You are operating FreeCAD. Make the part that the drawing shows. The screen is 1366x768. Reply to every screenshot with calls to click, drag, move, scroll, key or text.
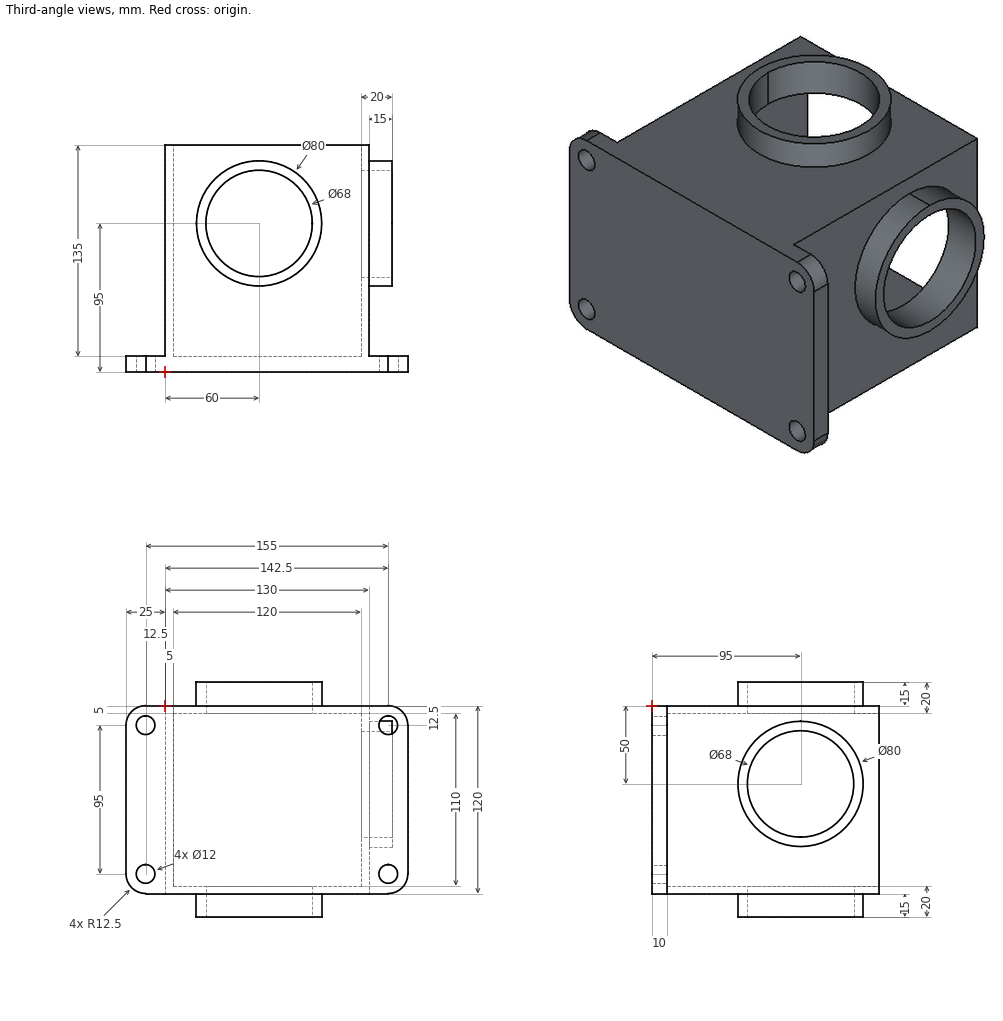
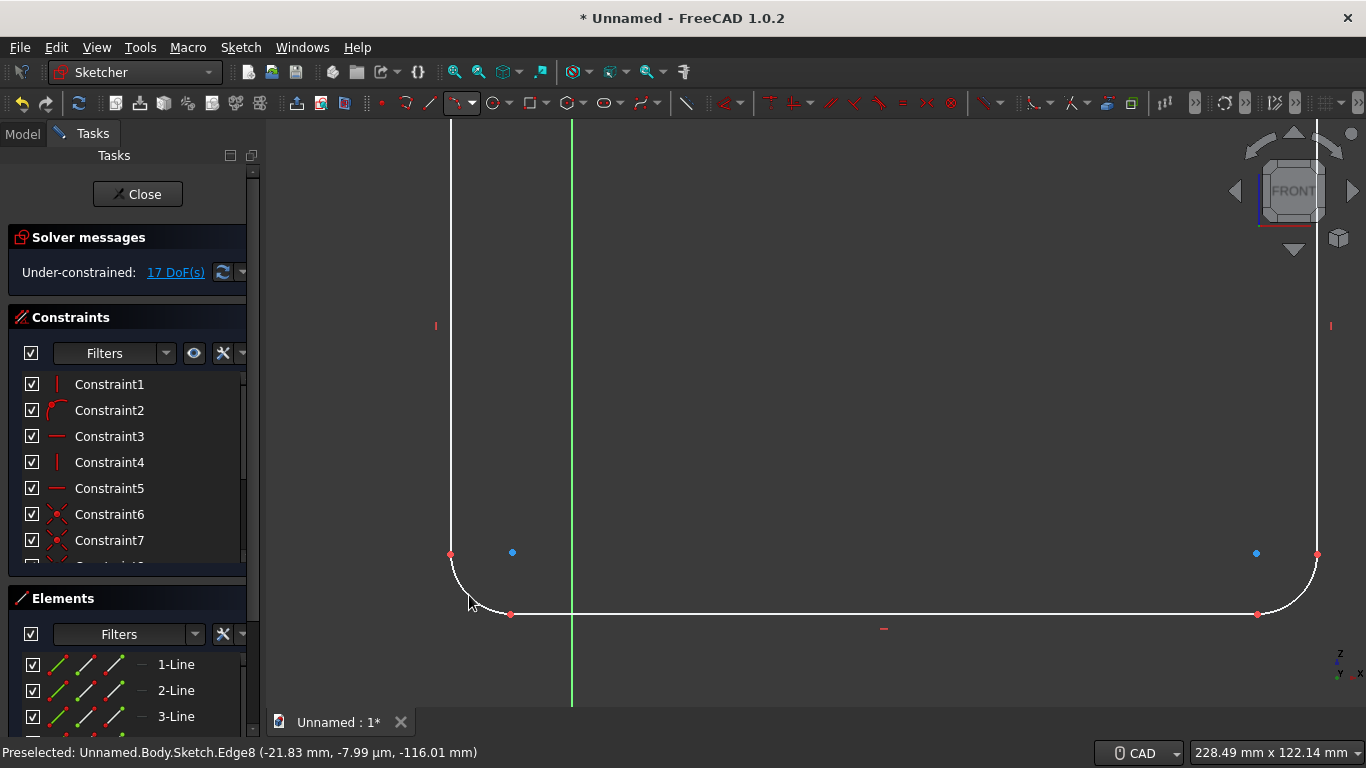
click(451, 417)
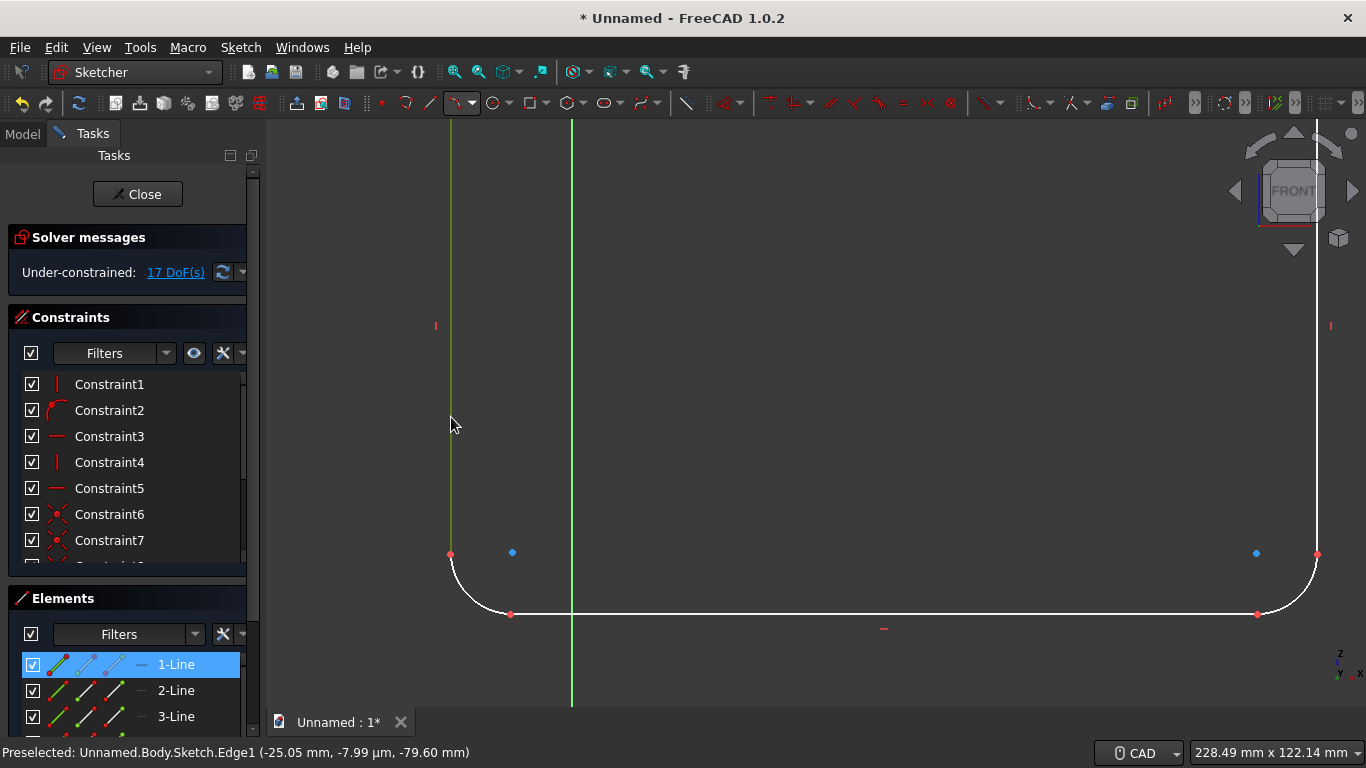
scroll(469, 595, down, 2)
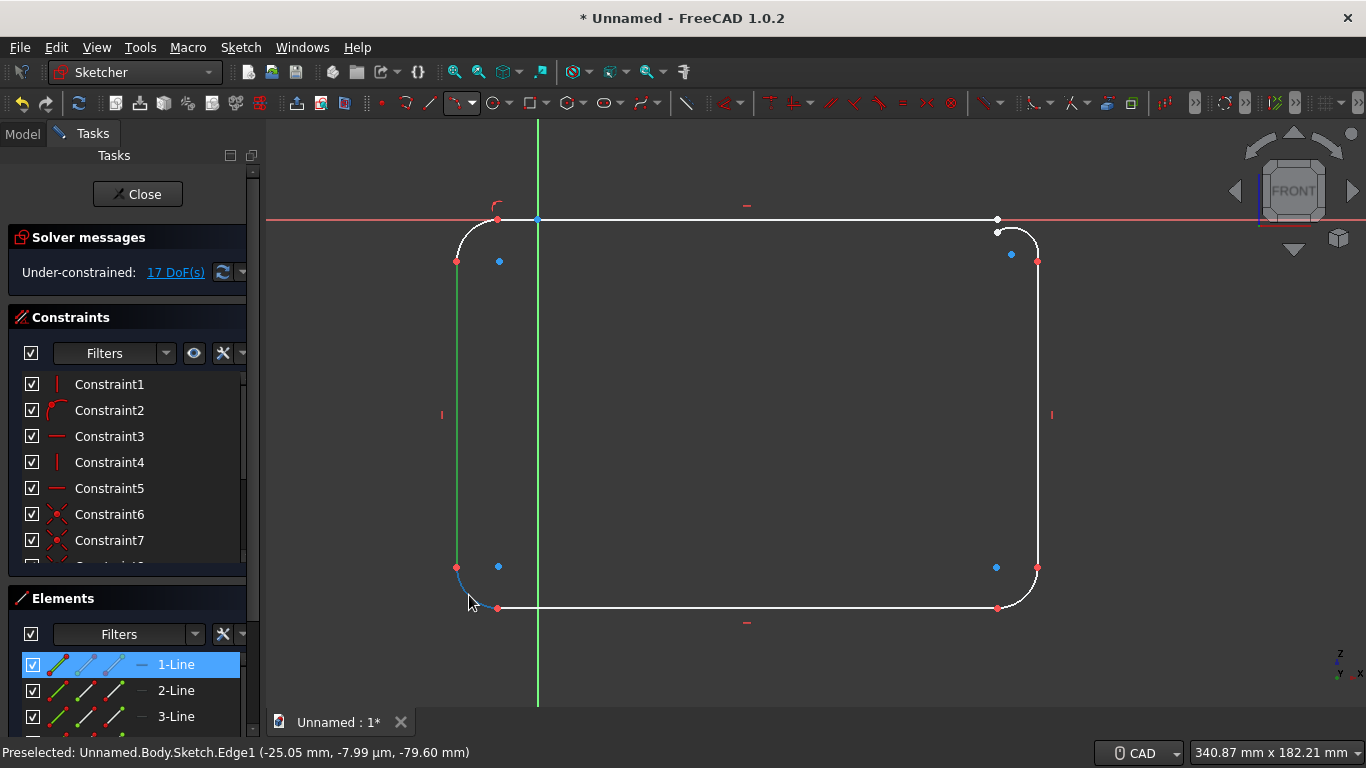
click(462, 243)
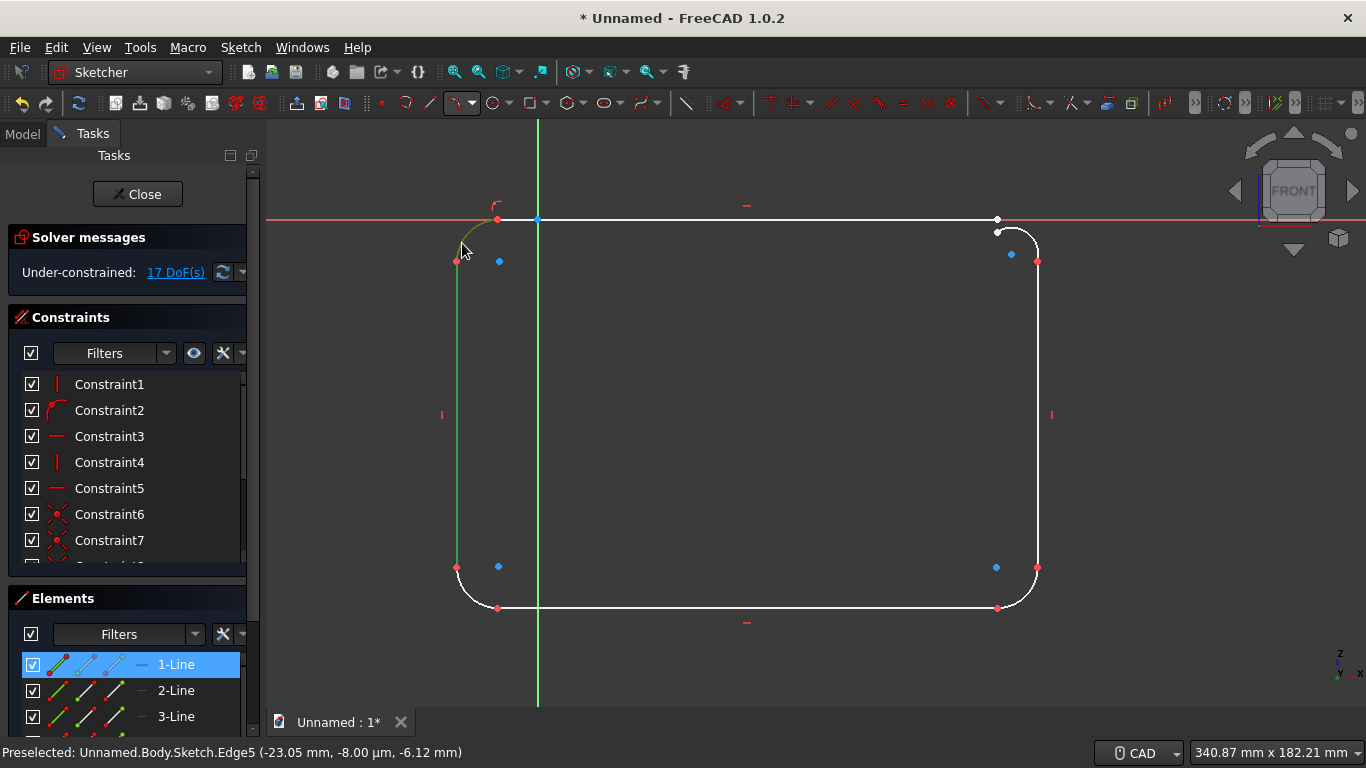
click(880, 104)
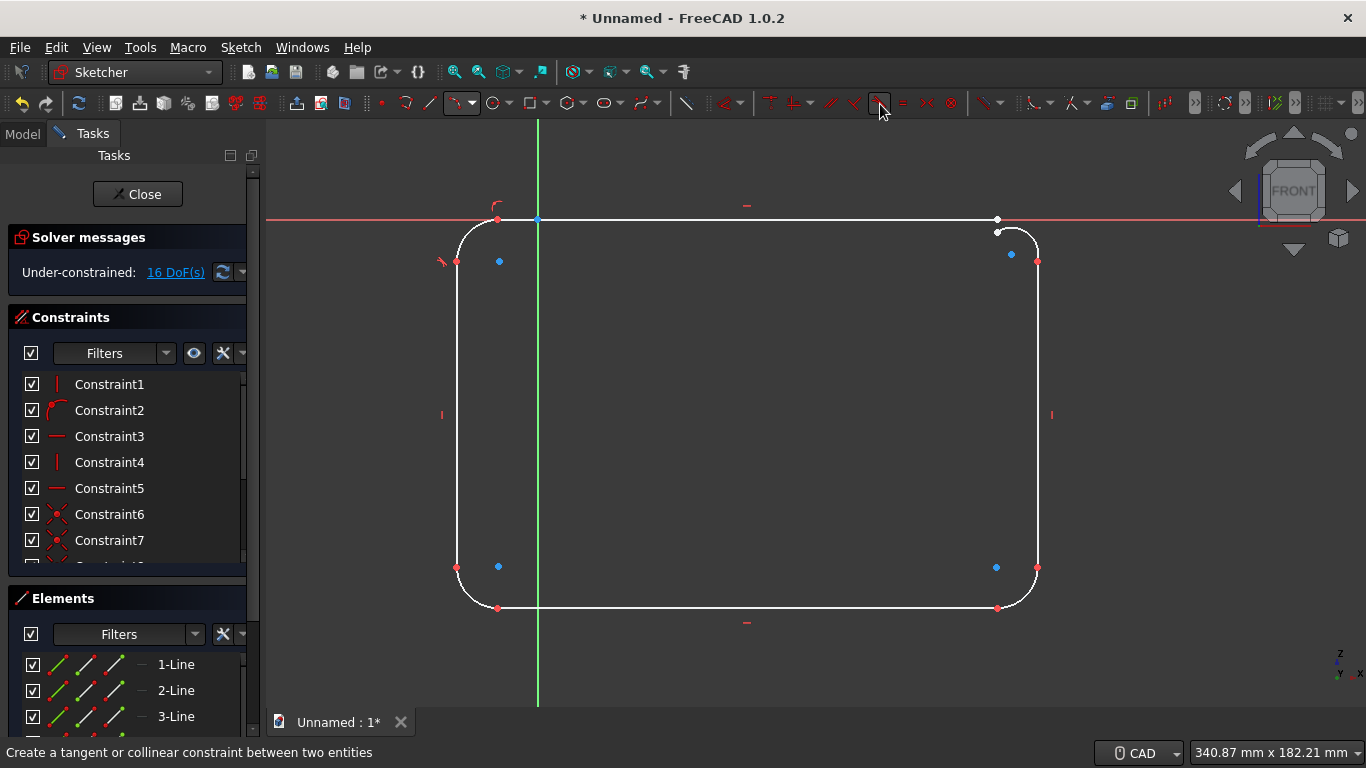
click(457, 476)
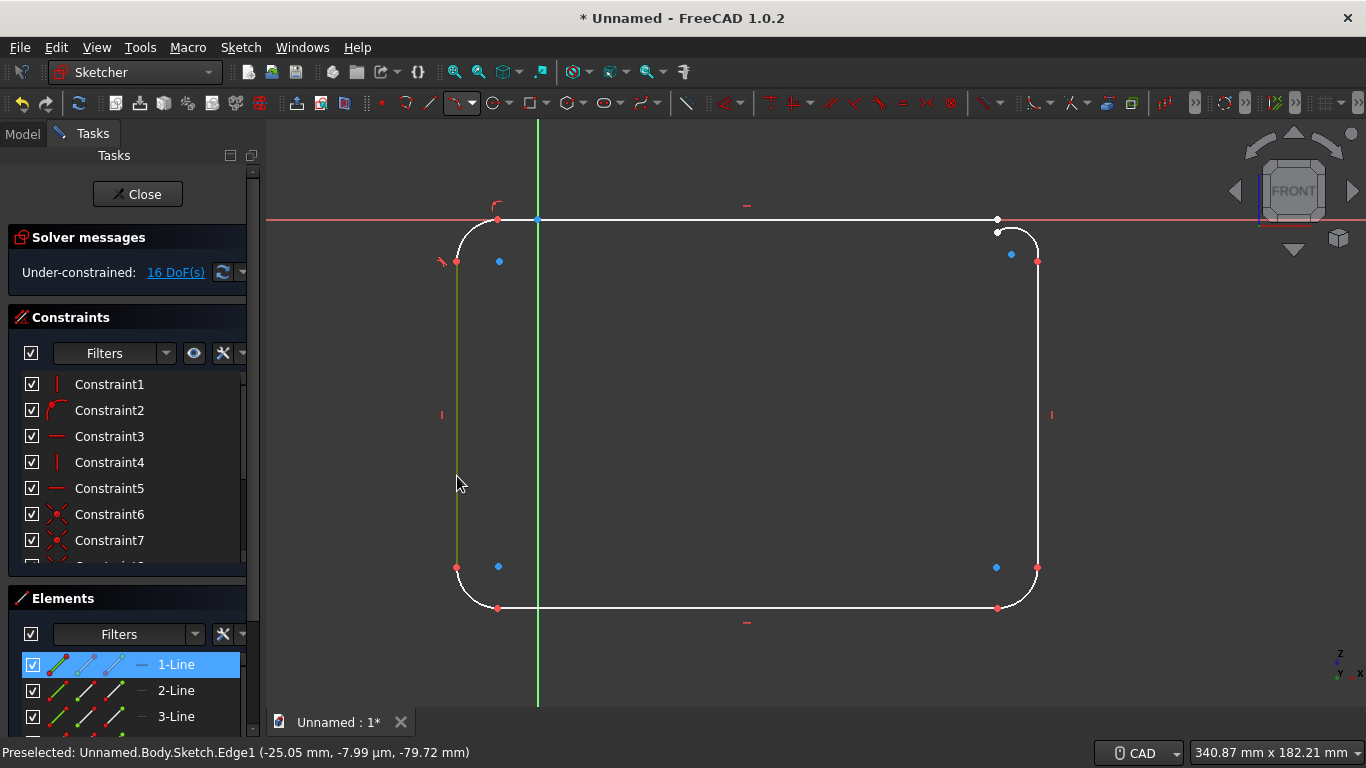
click(462, 586)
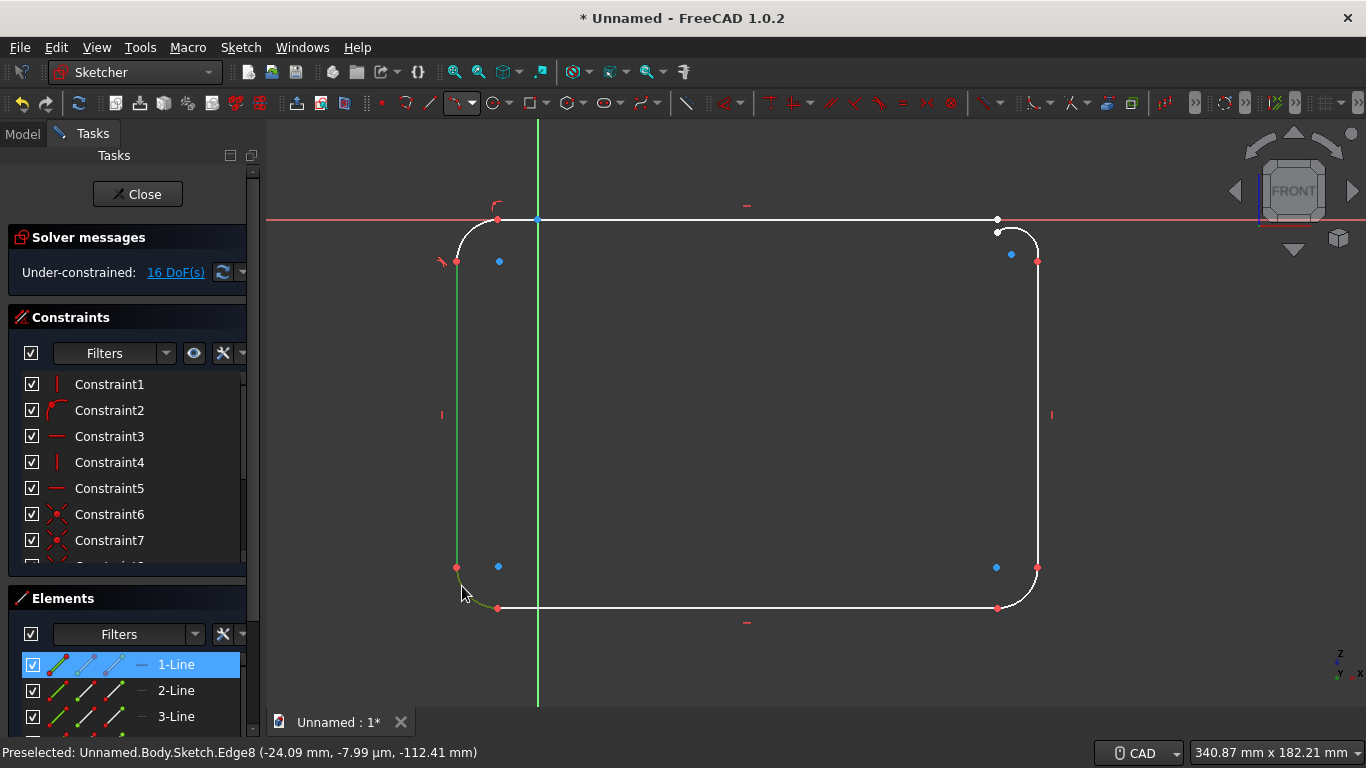
key(t)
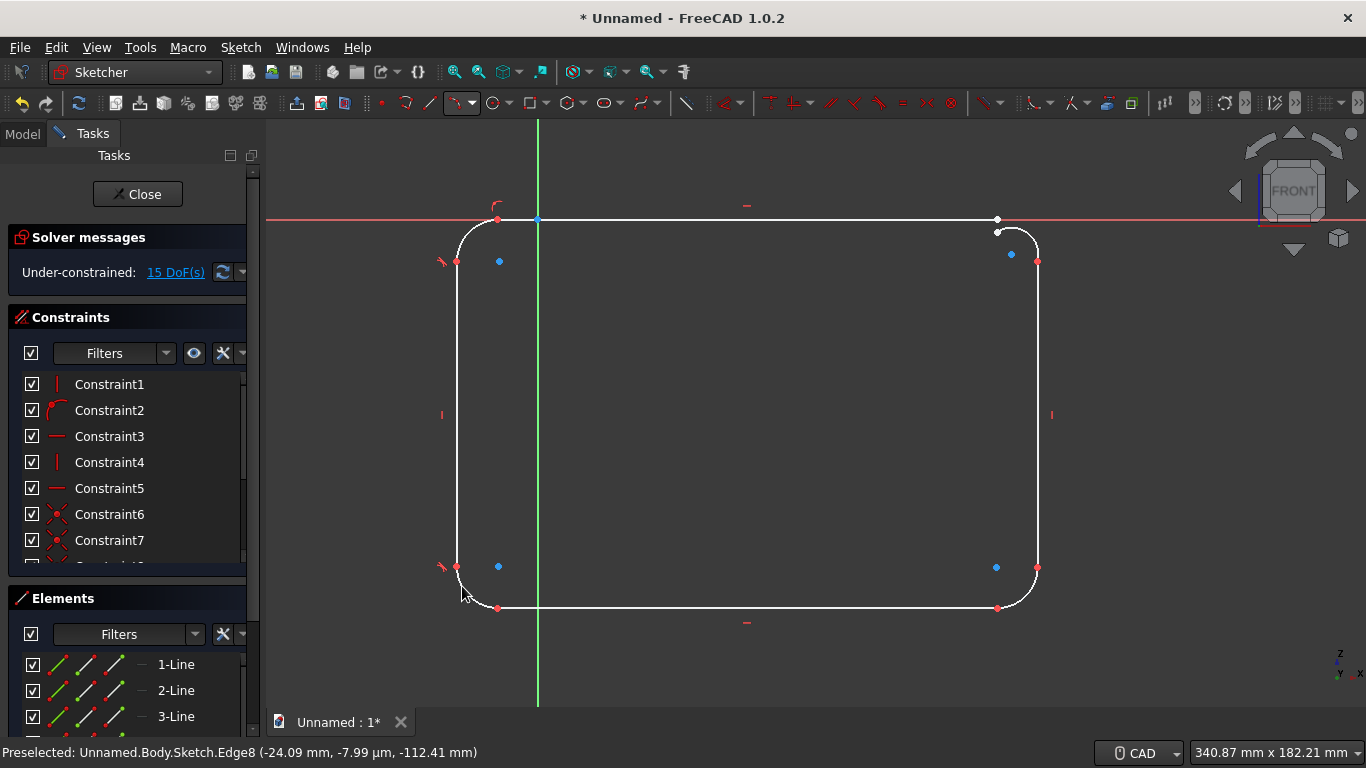
click(647, 220)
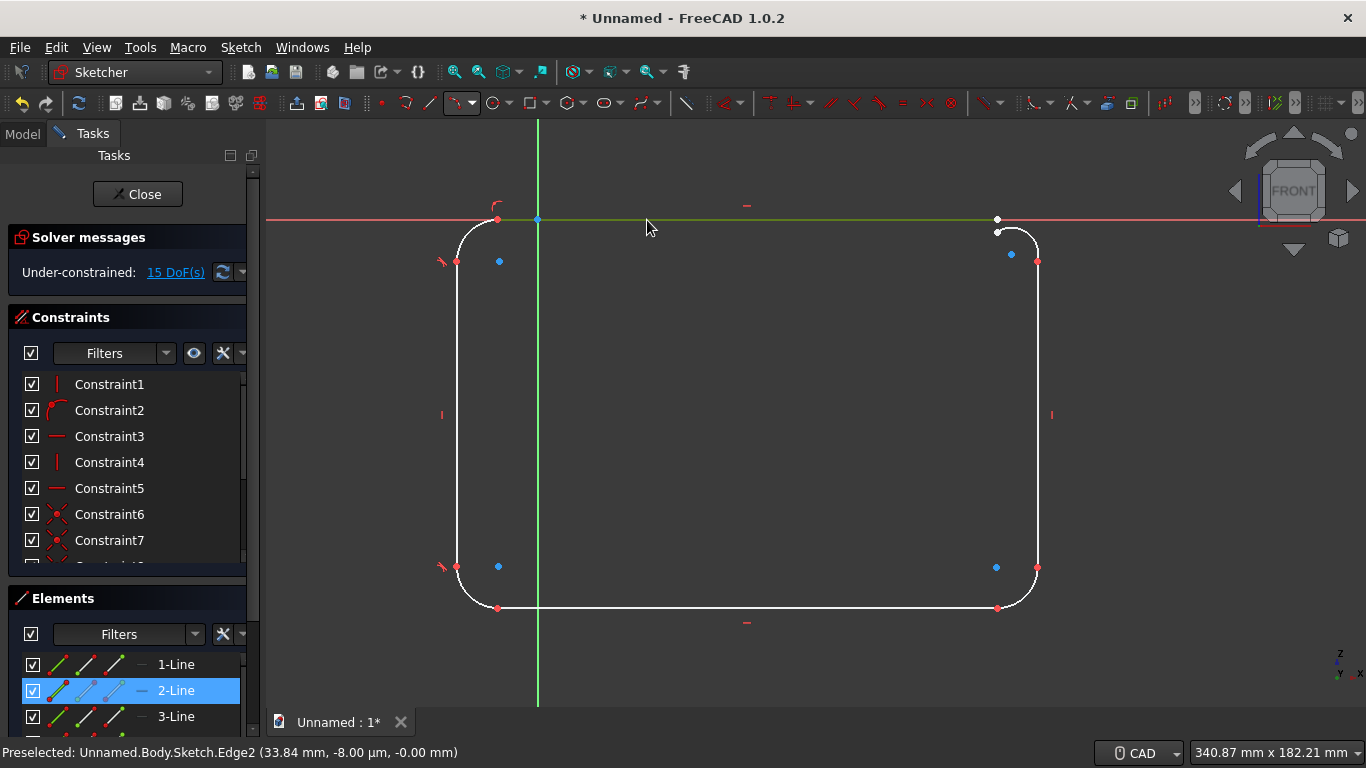
click(461, 243)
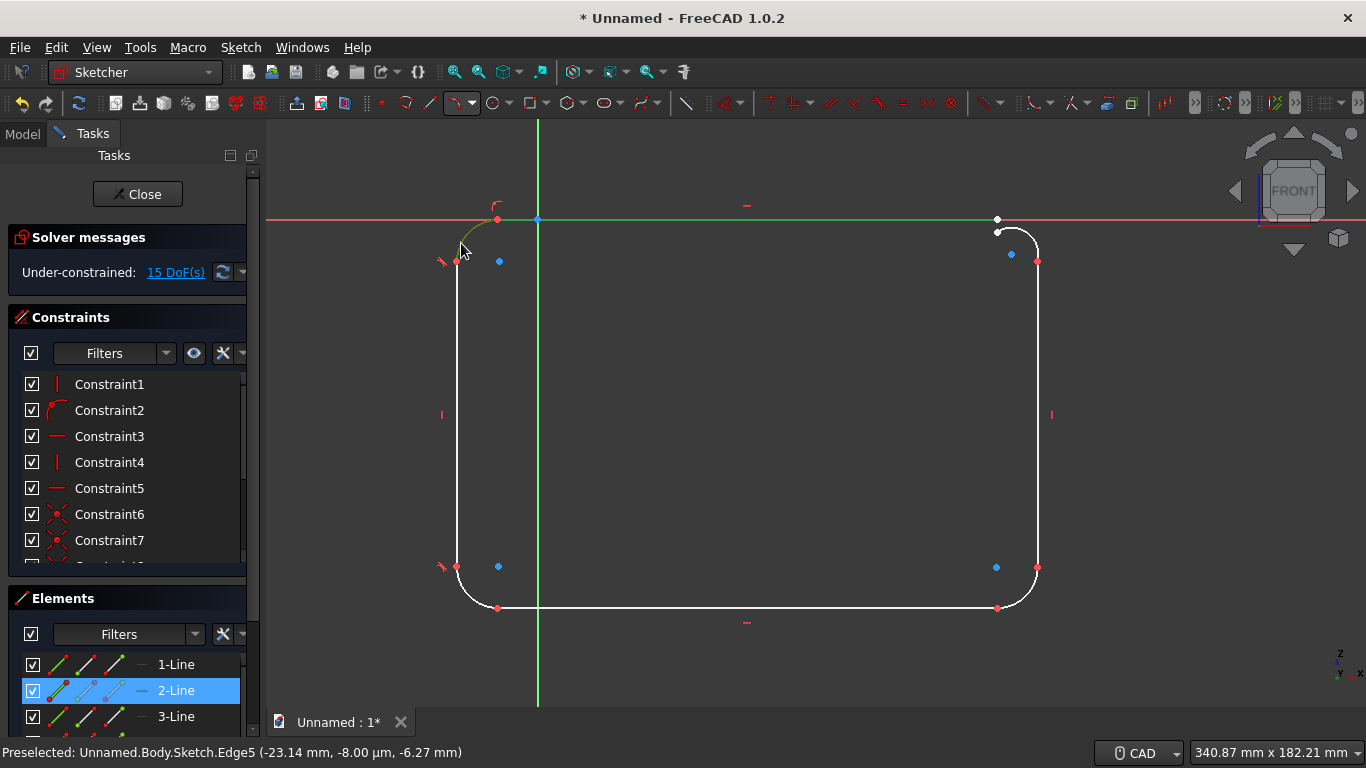
key(t)